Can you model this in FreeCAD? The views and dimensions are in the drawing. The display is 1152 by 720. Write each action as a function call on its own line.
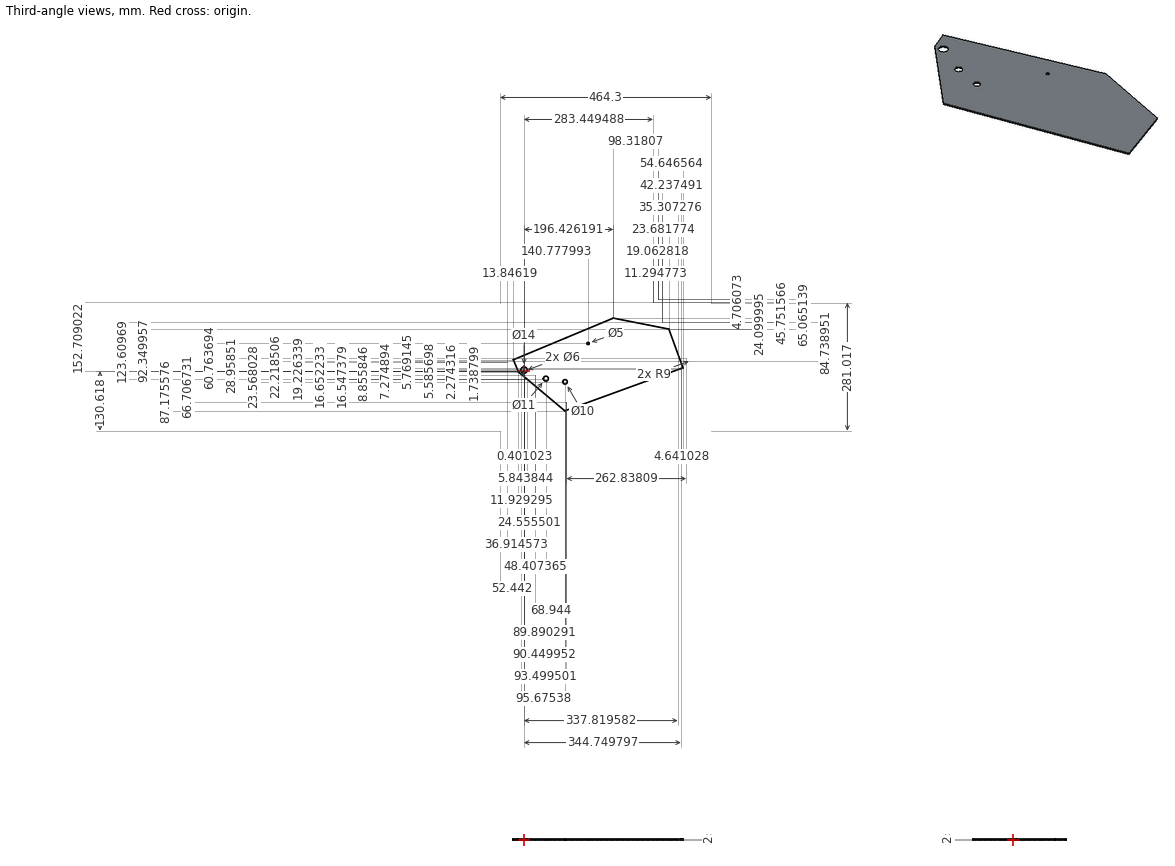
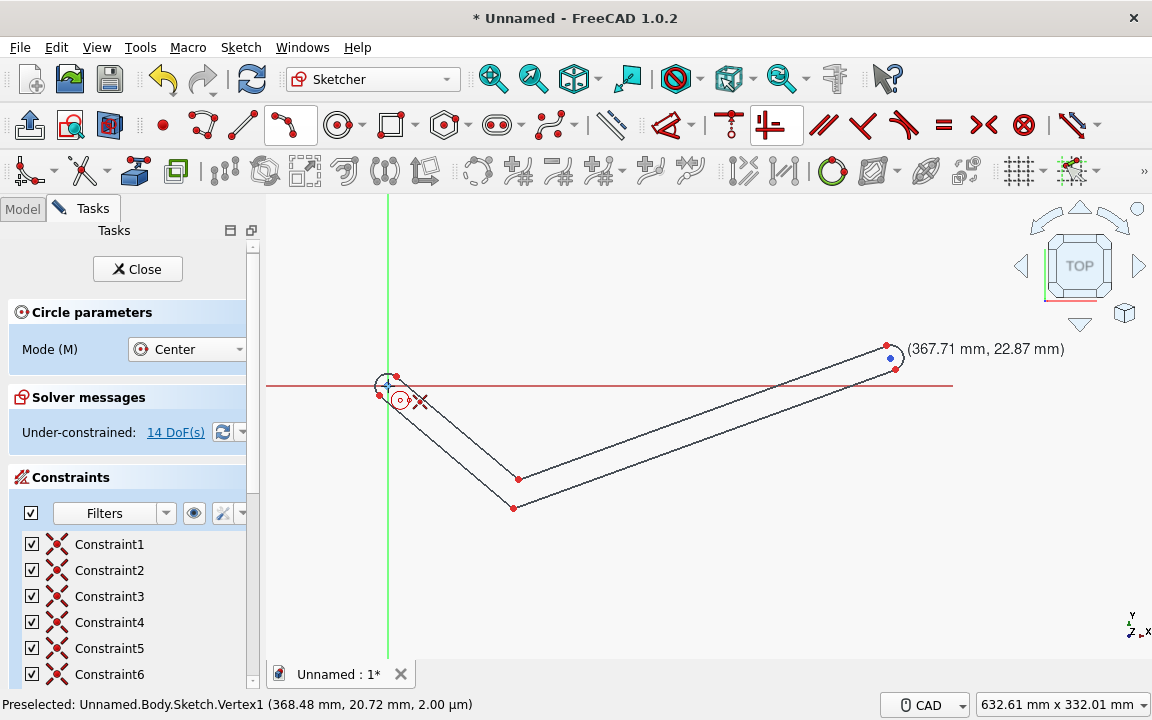
scroll(388, 386, up, 2)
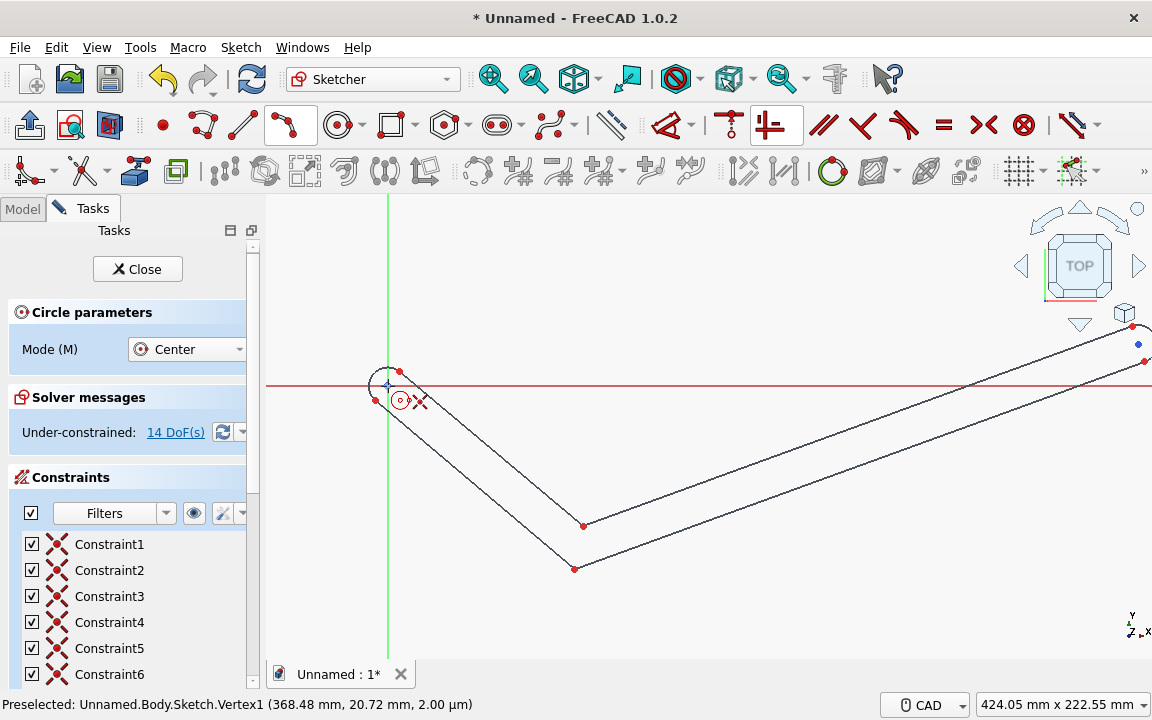
click(388, 386)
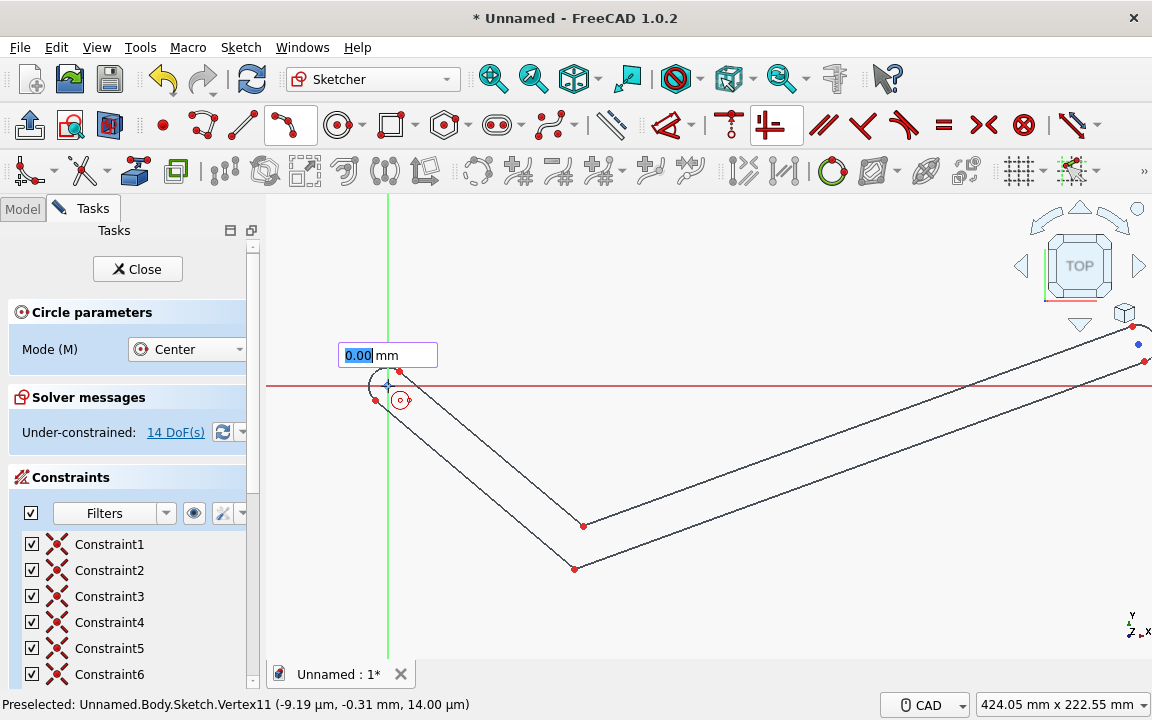
scroll(392, 381, up, 7)
move(393, 381)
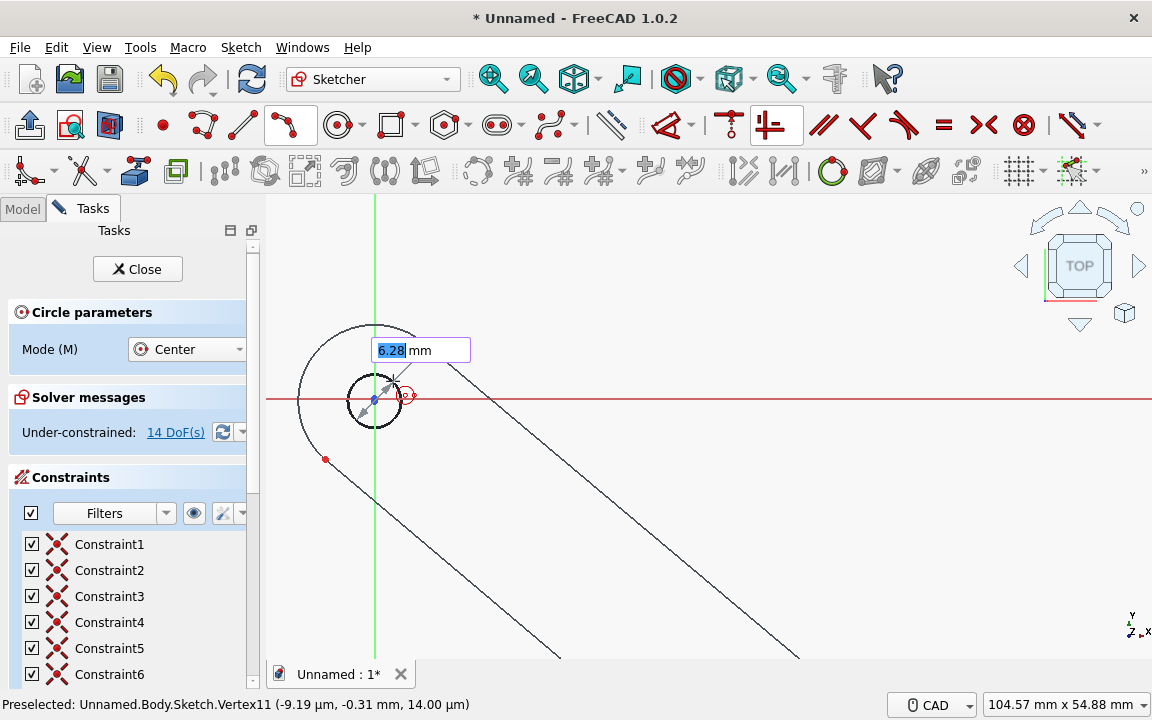
text(6)
key(Return)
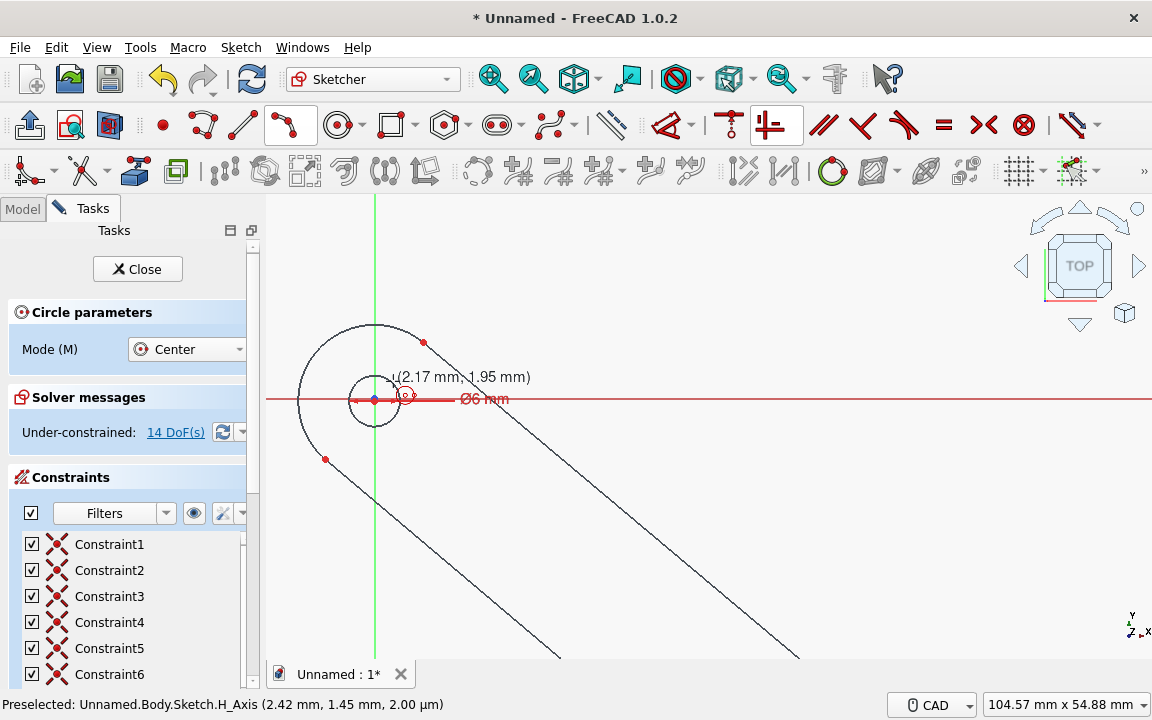
scroll(390, 383, down, 9)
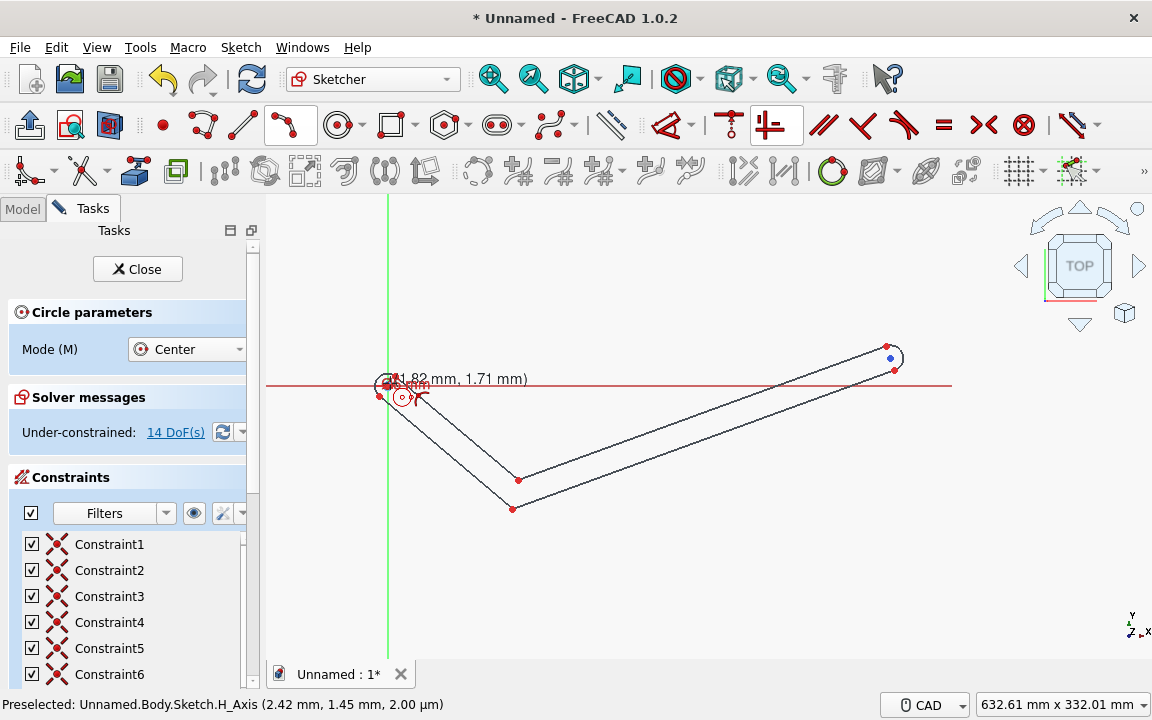
scroll(891, 357, up, 9)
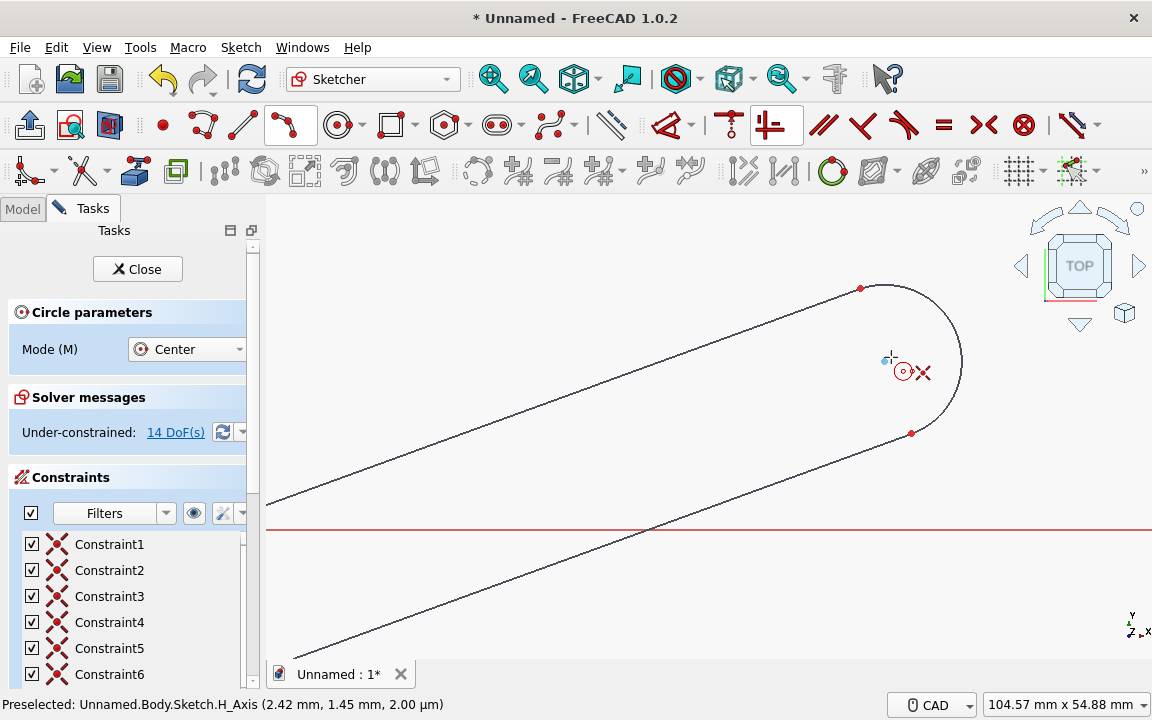
scroll(892, 357, down, 9)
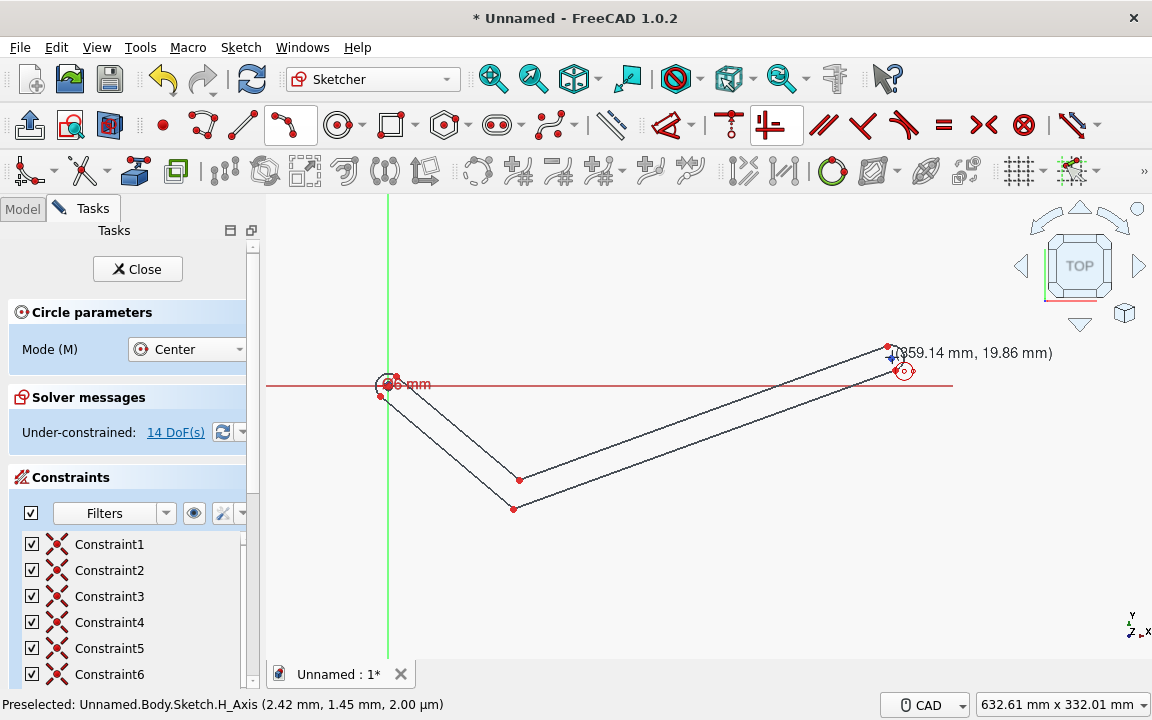
scroll(892, 357, up, 2)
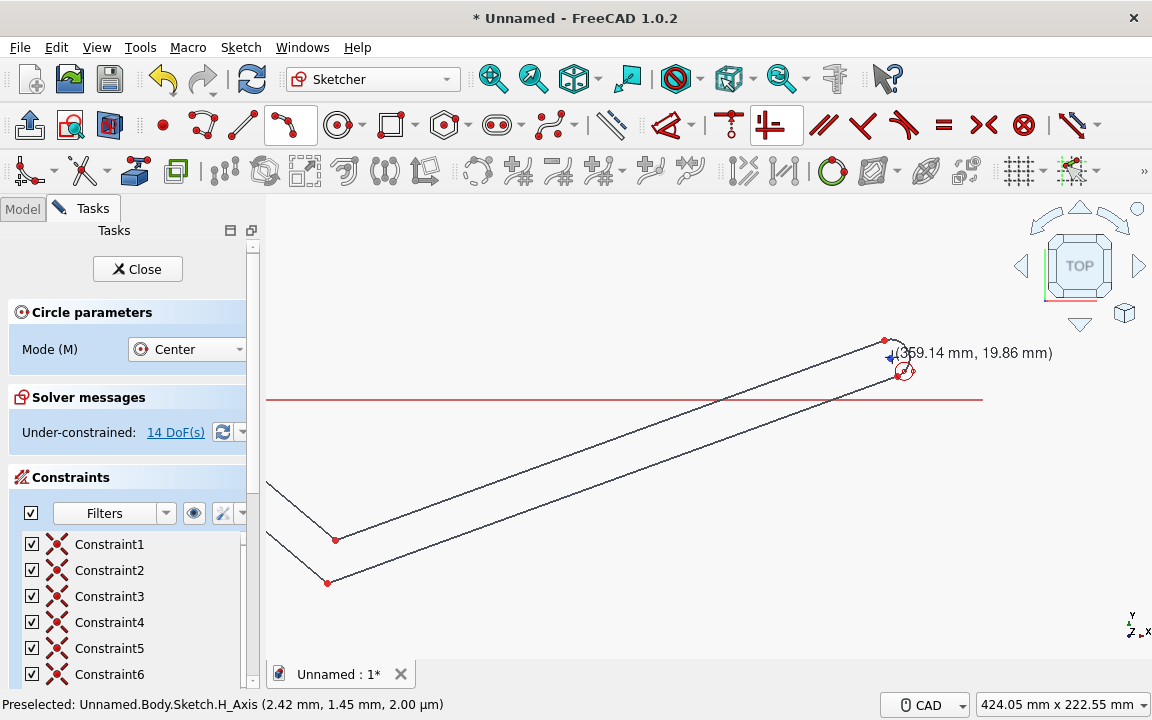
click(891, 357)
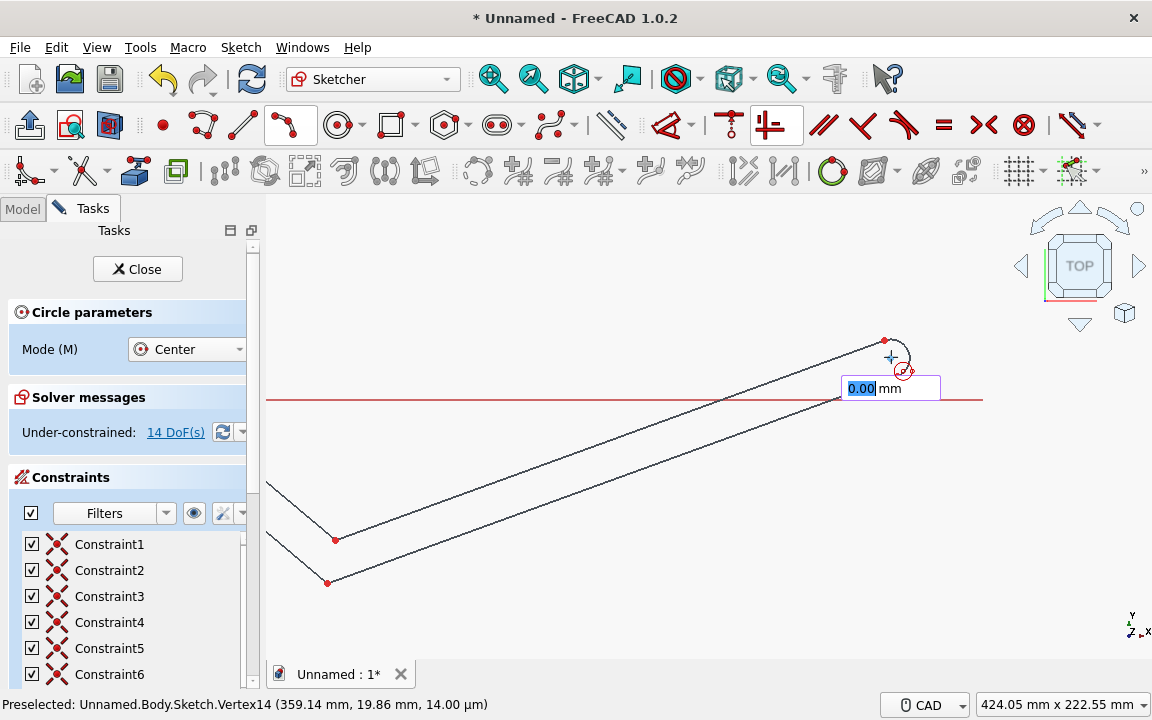
scroll(897, 355, up, 5)
move(896, 354)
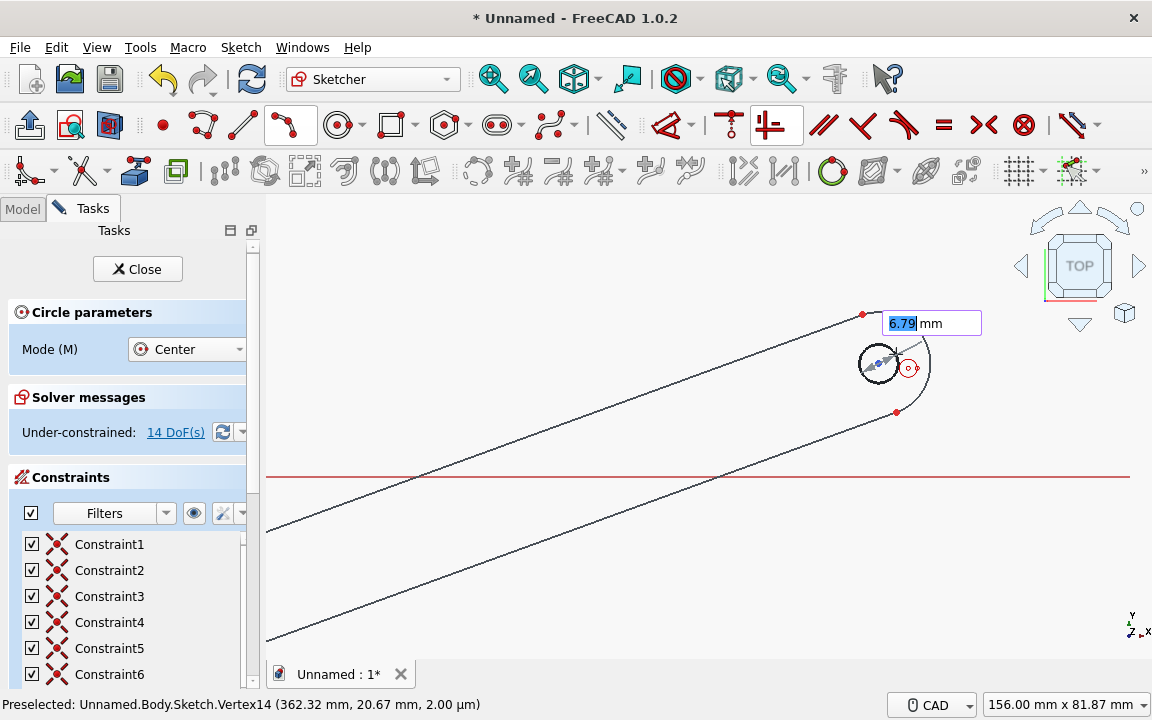
text(6)
key(Return)
key(Escape)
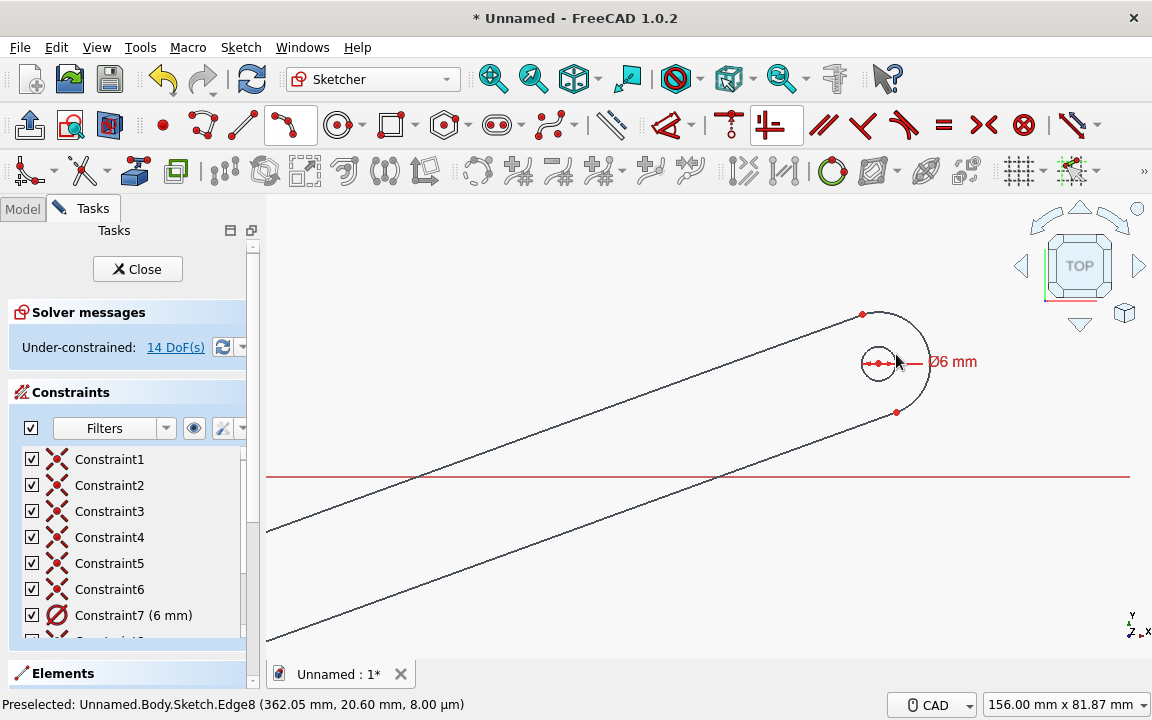
scroll(895, 356, down, 7)